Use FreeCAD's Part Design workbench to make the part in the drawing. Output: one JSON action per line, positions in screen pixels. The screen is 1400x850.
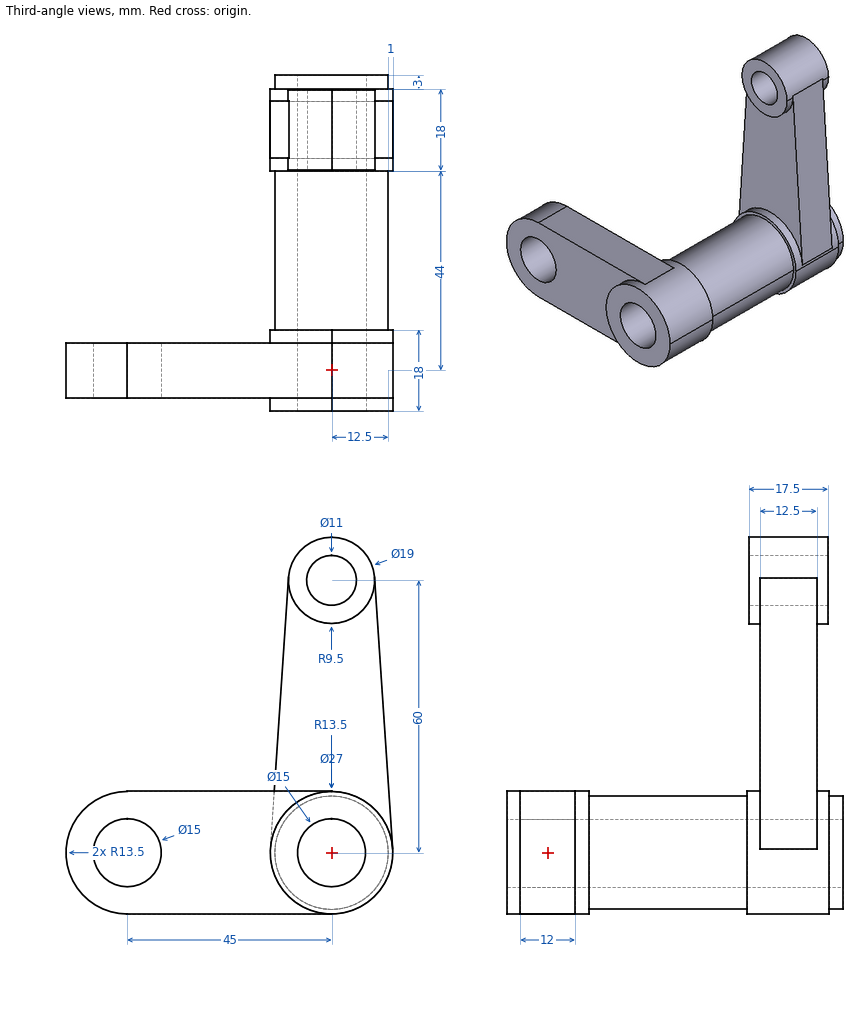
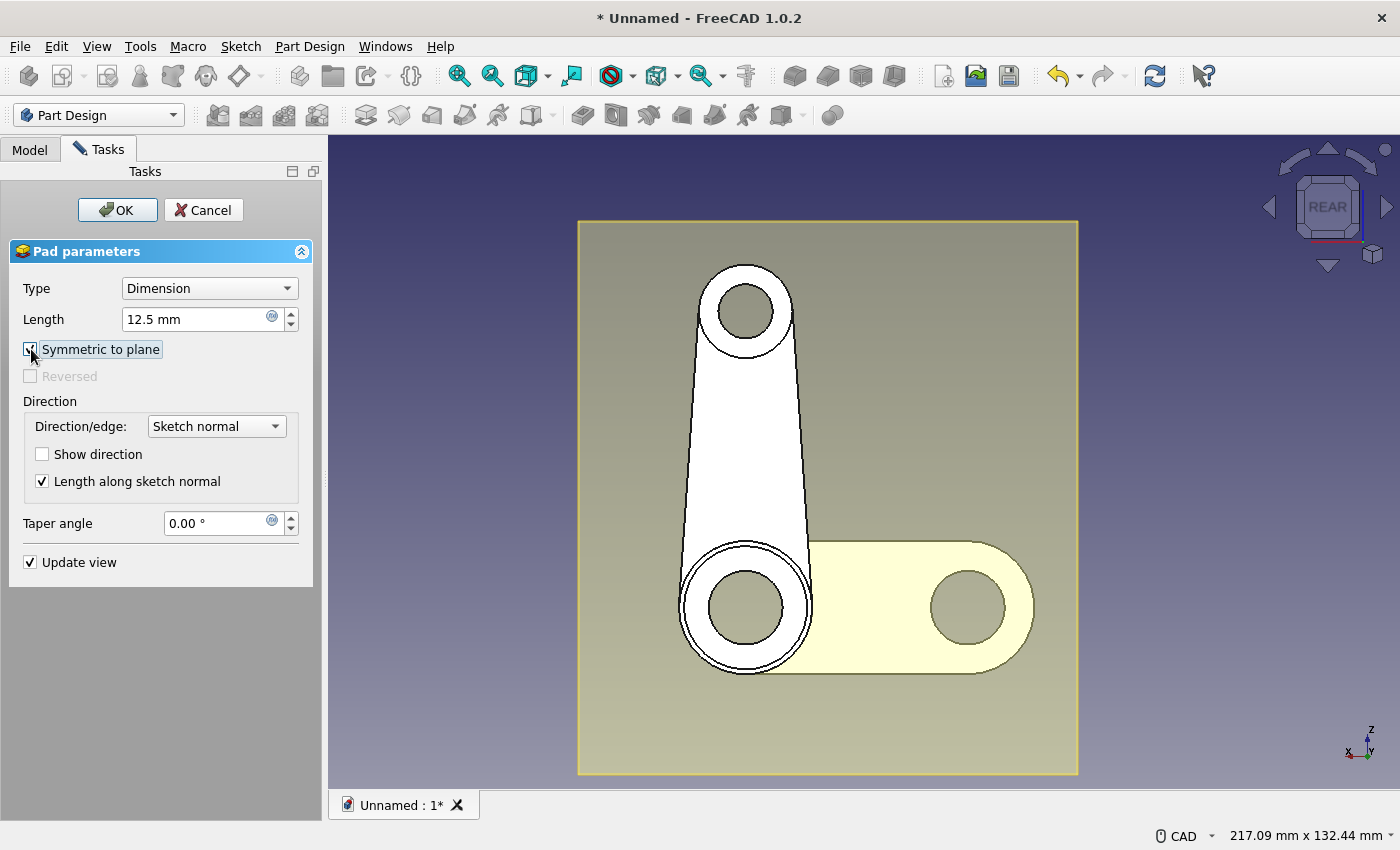
{"action": "left_click", "coordinate": [118, 210]}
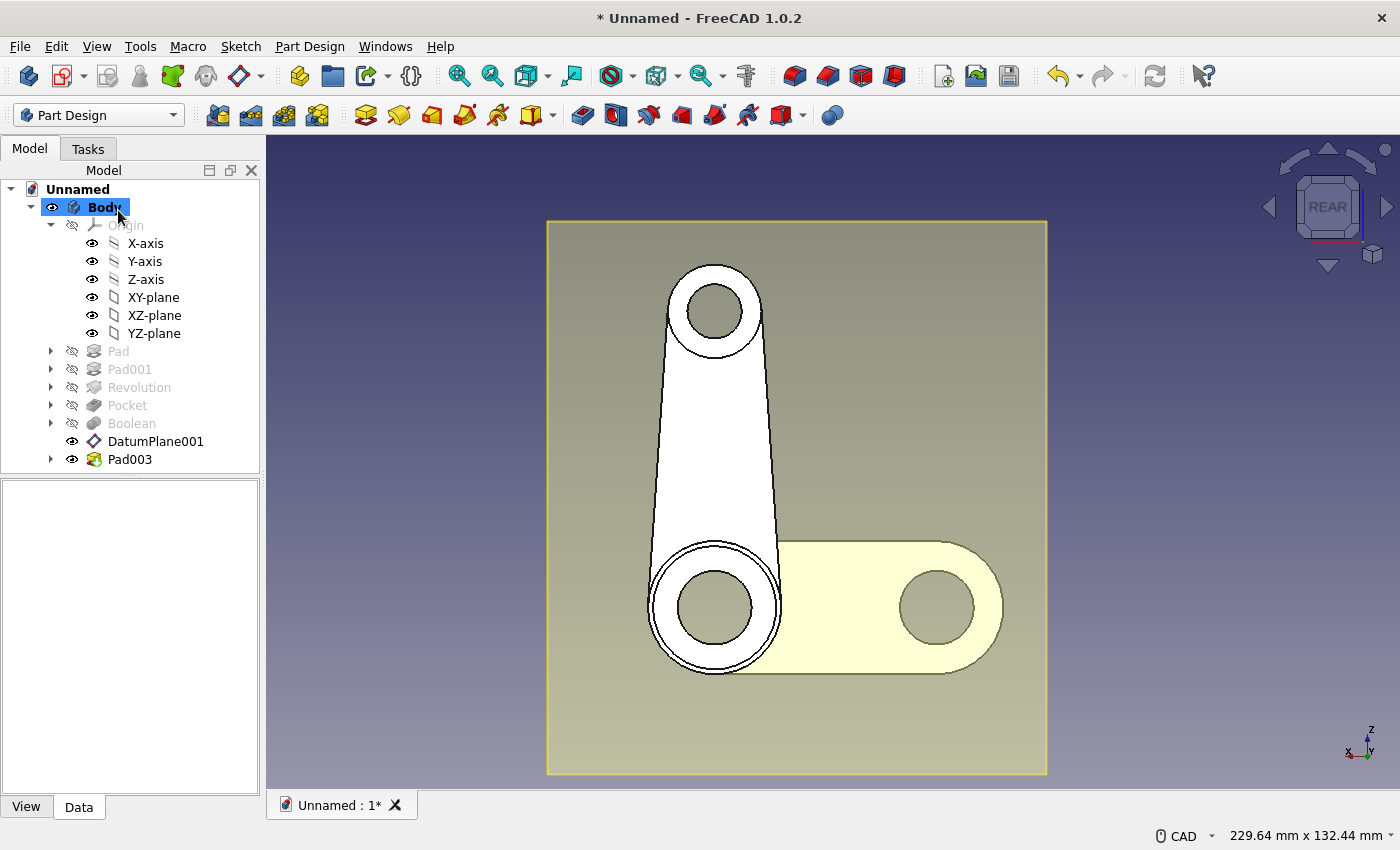
{"action": "left_click", "coordinate": [117, 441]}
{"action": "key", "text": "space"}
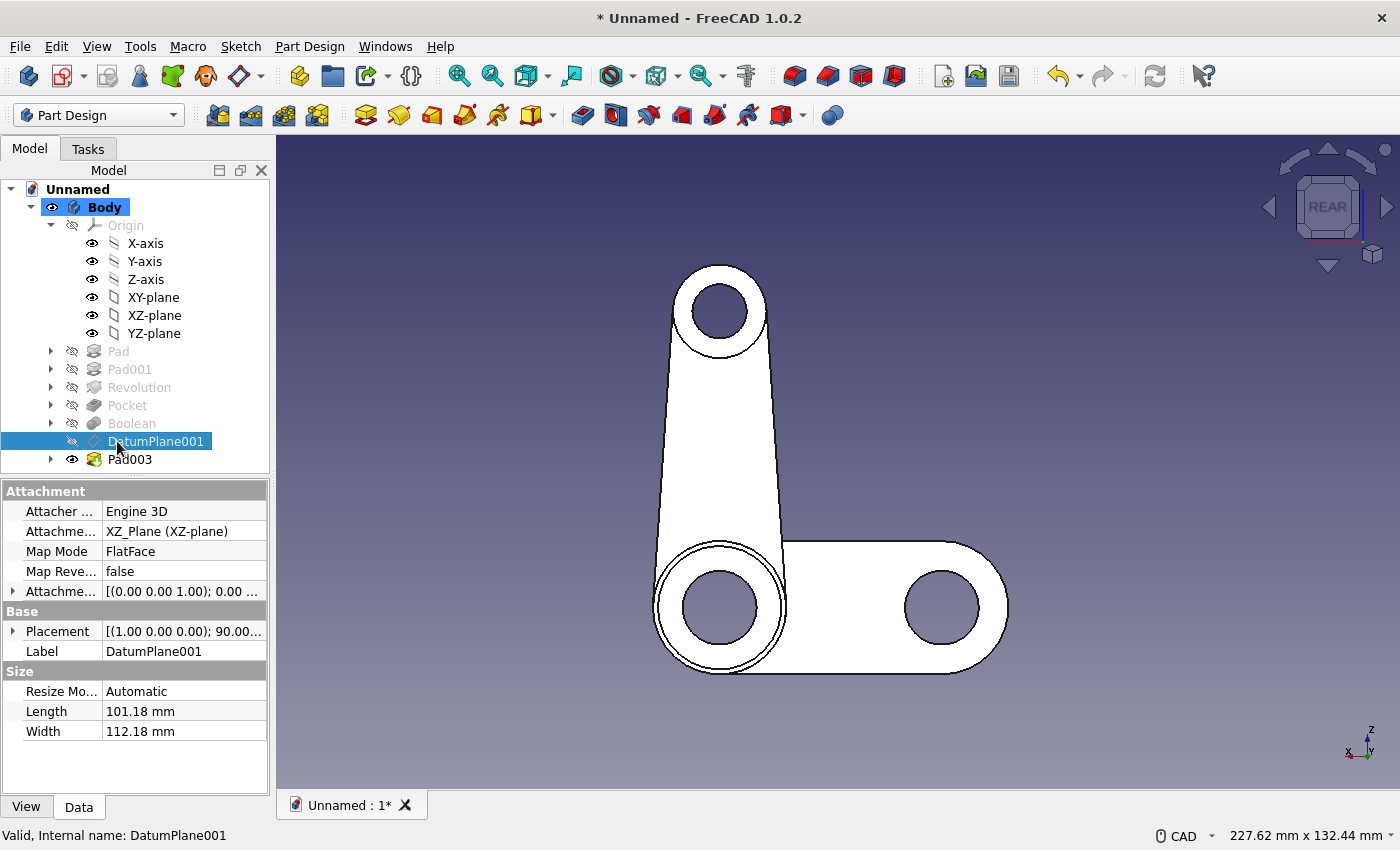
{"action": "key", "text": "0"}